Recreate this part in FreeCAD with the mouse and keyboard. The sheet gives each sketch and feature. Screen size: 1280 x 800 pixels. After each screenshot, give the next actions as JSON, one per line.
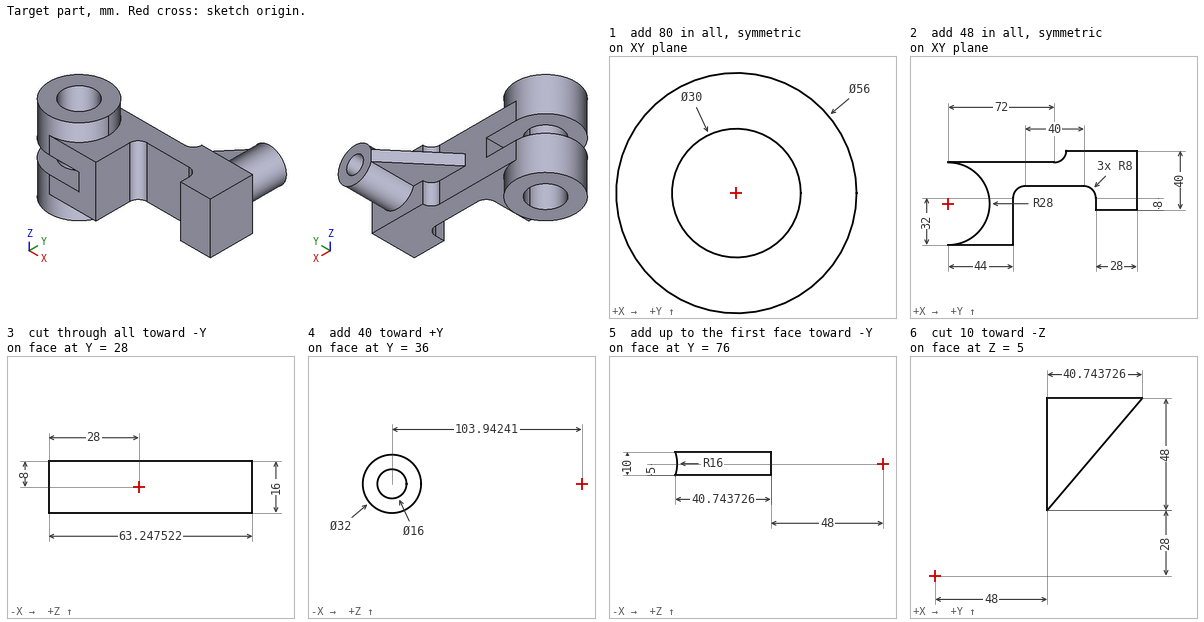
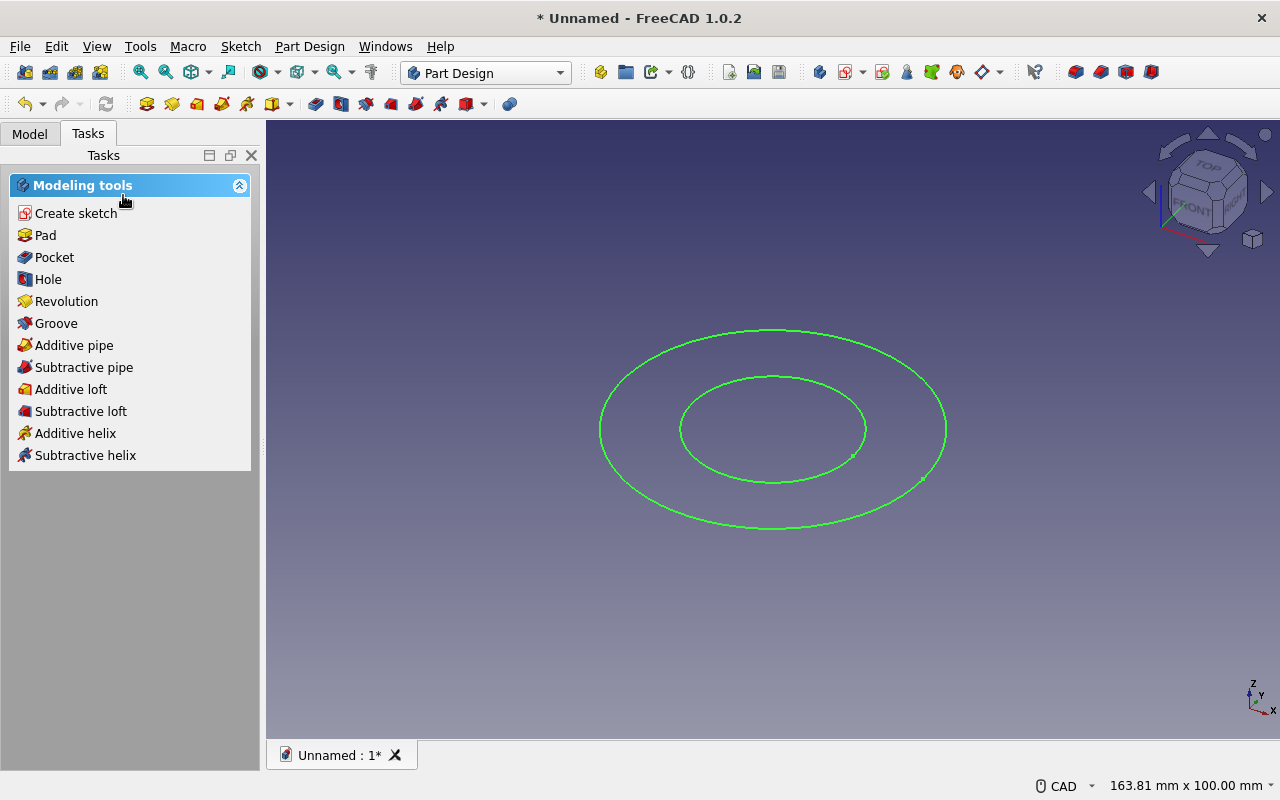
{"action": "left_click", "coordinate": [147, 104]}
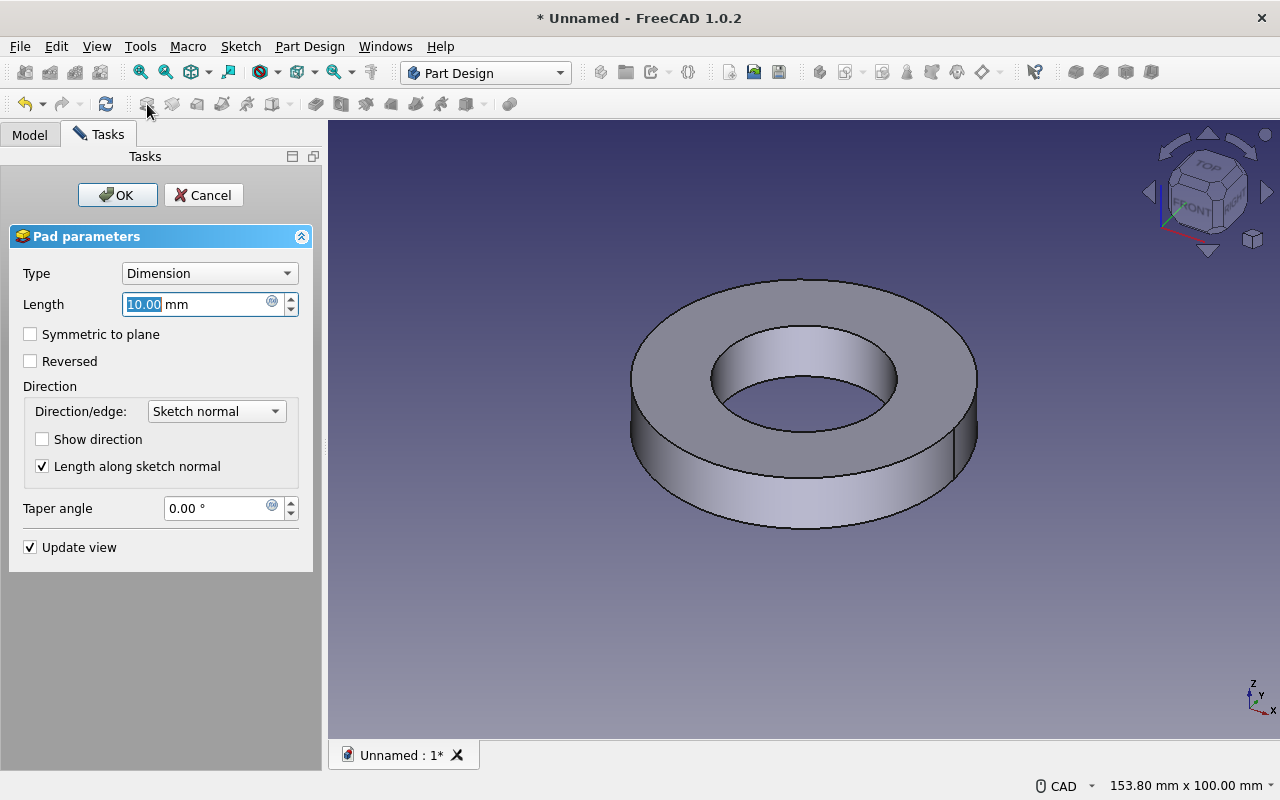
{"action": "type", "text": "80"}
{"action": "key", "text": "Tab"}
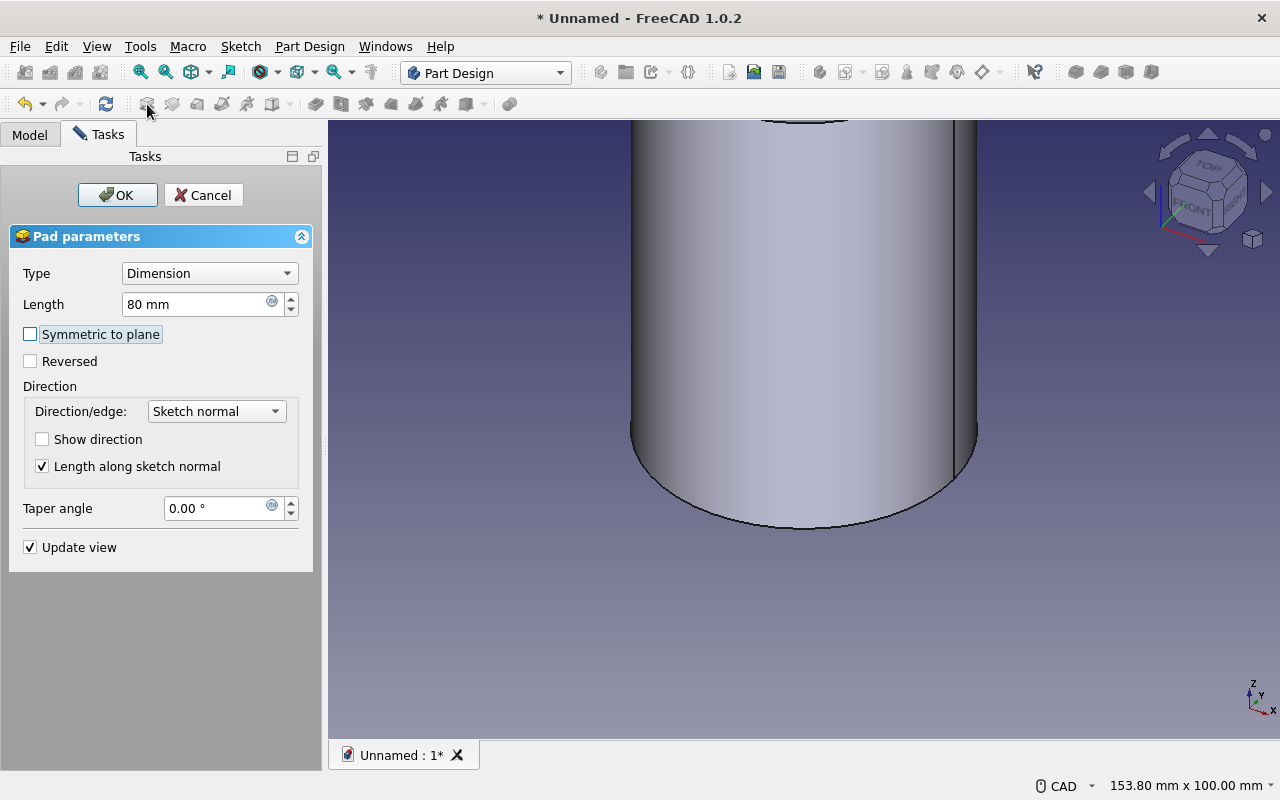
{"action": "left_click", "coordinate": [31, 334]}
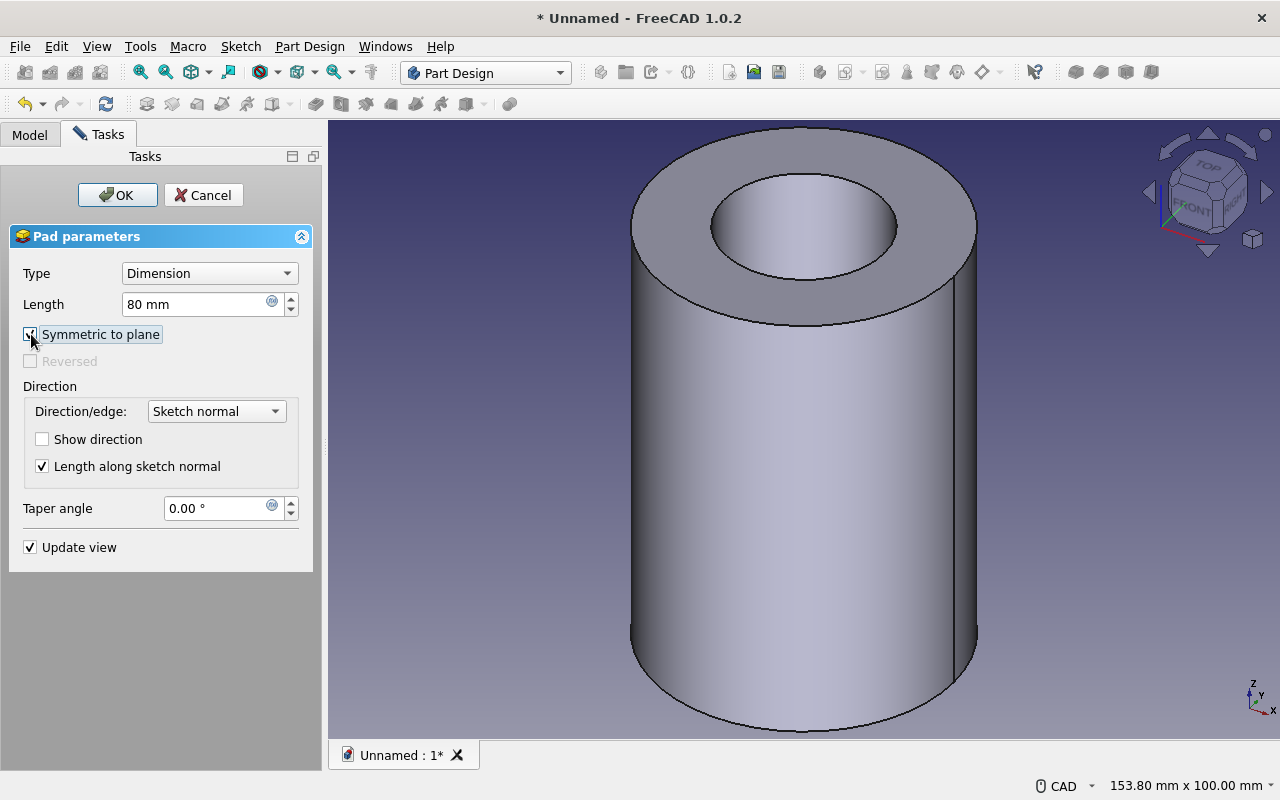
{"action": "left_click", "coordinate": [118, 195]}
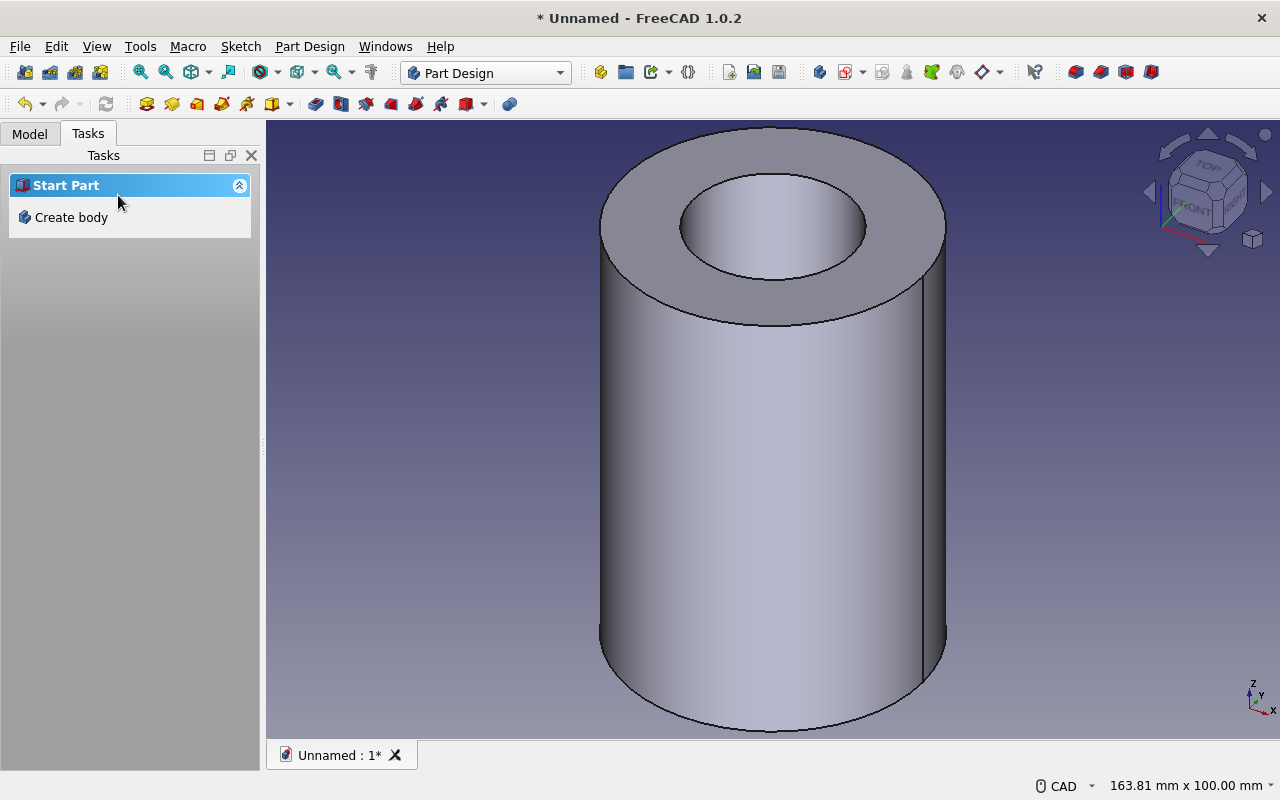
{"action": "key", "text": "v f"}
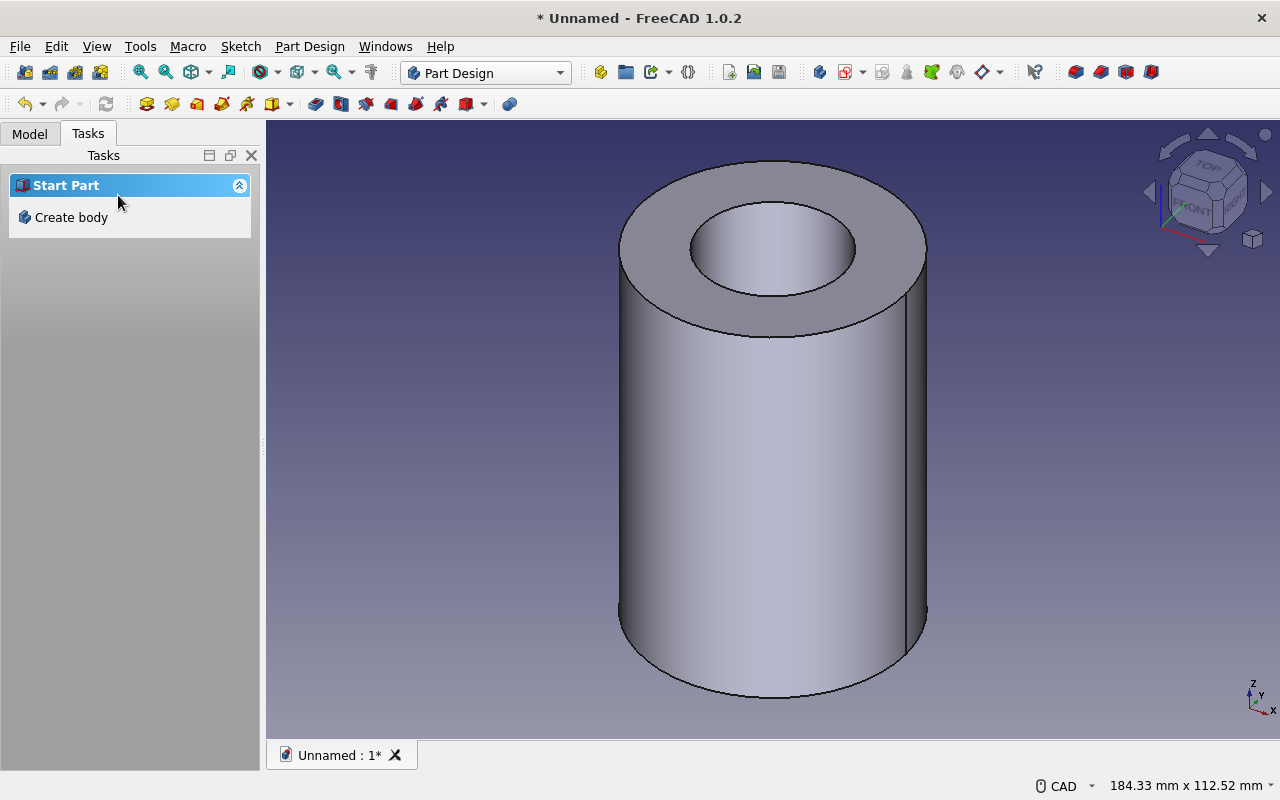
{"action": "left_click", "coordinate": [844, 72]}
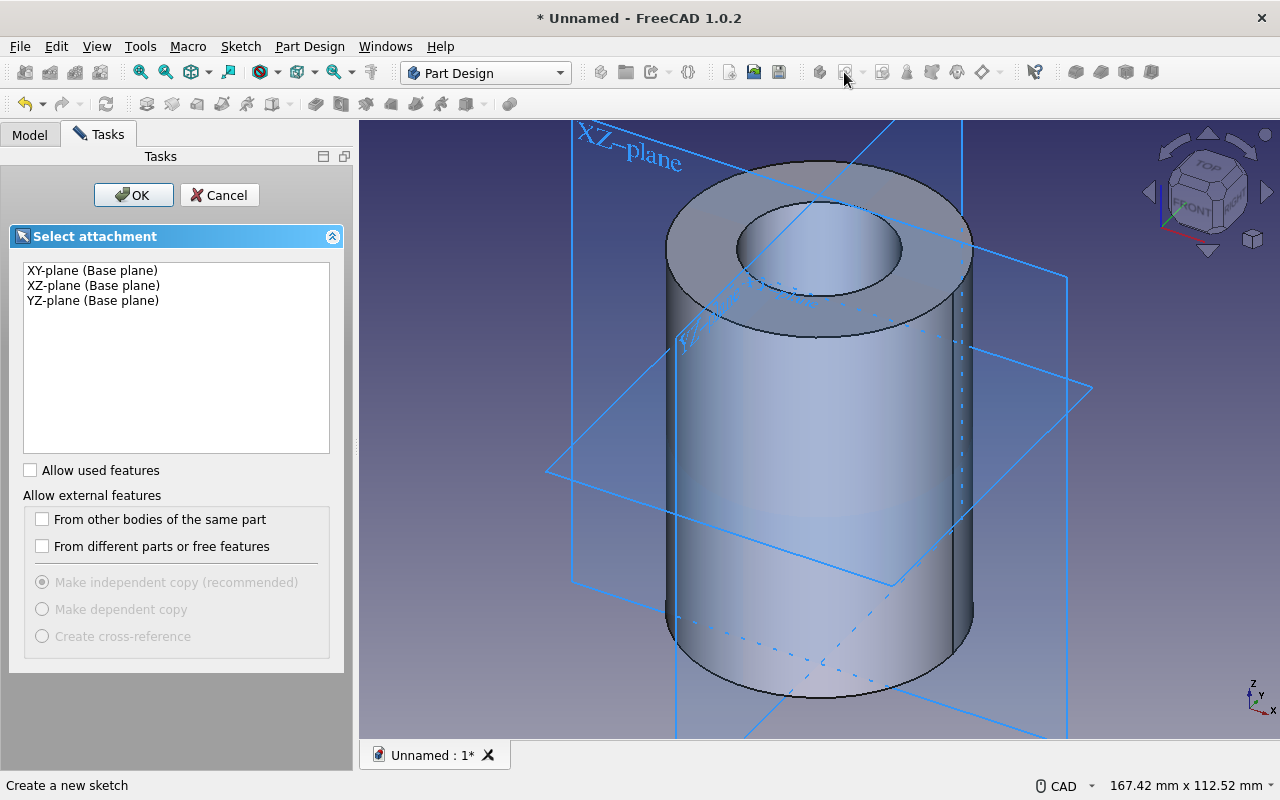
{"action": "left_click", "coordinate": [84, 270]}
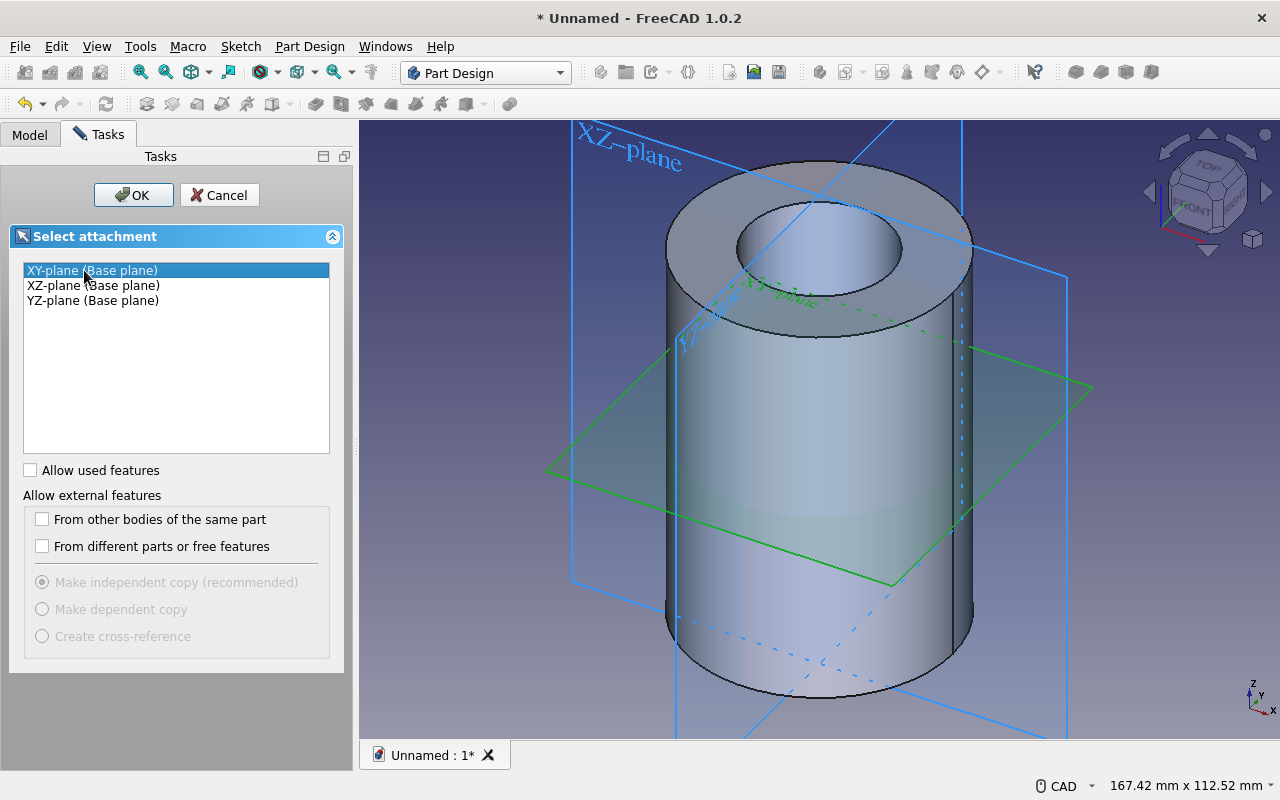
{"action": "left_click", "coordinate": [134, 195]}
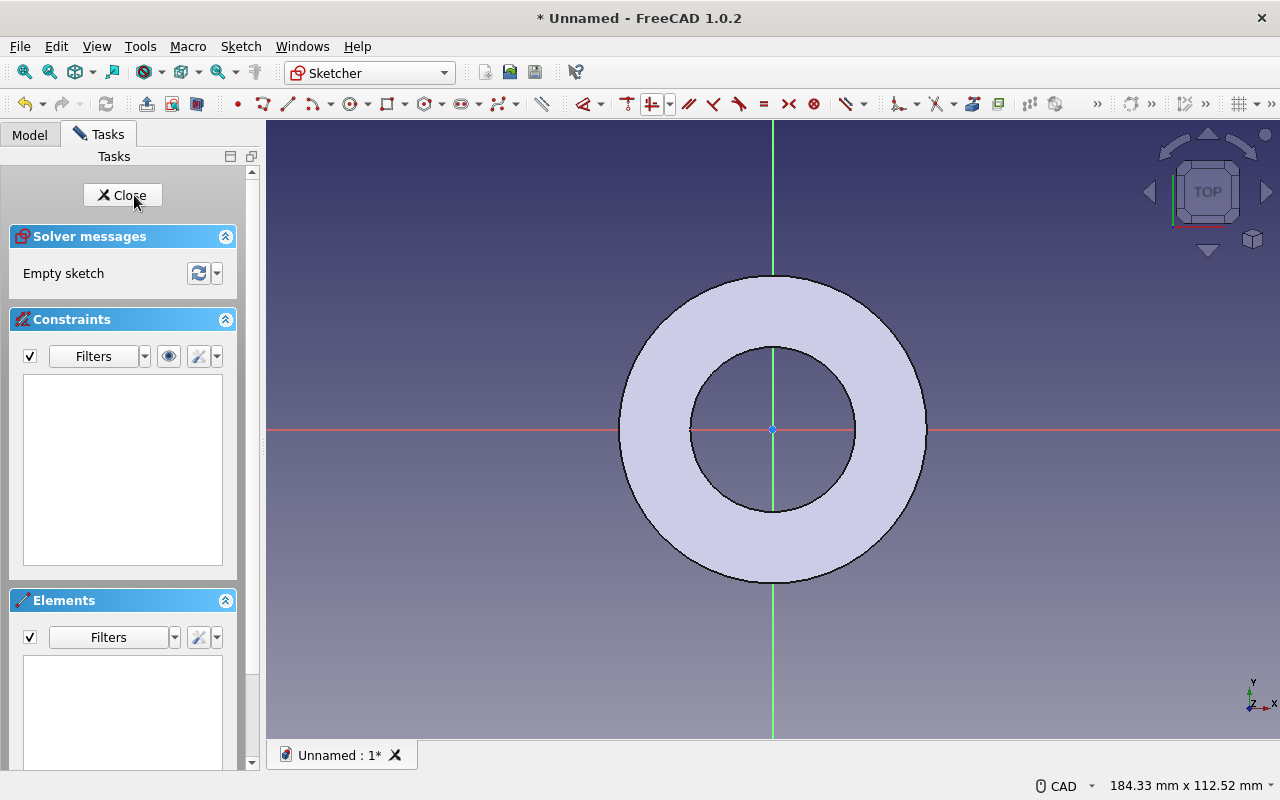
{"action": "key", "text": "q s"}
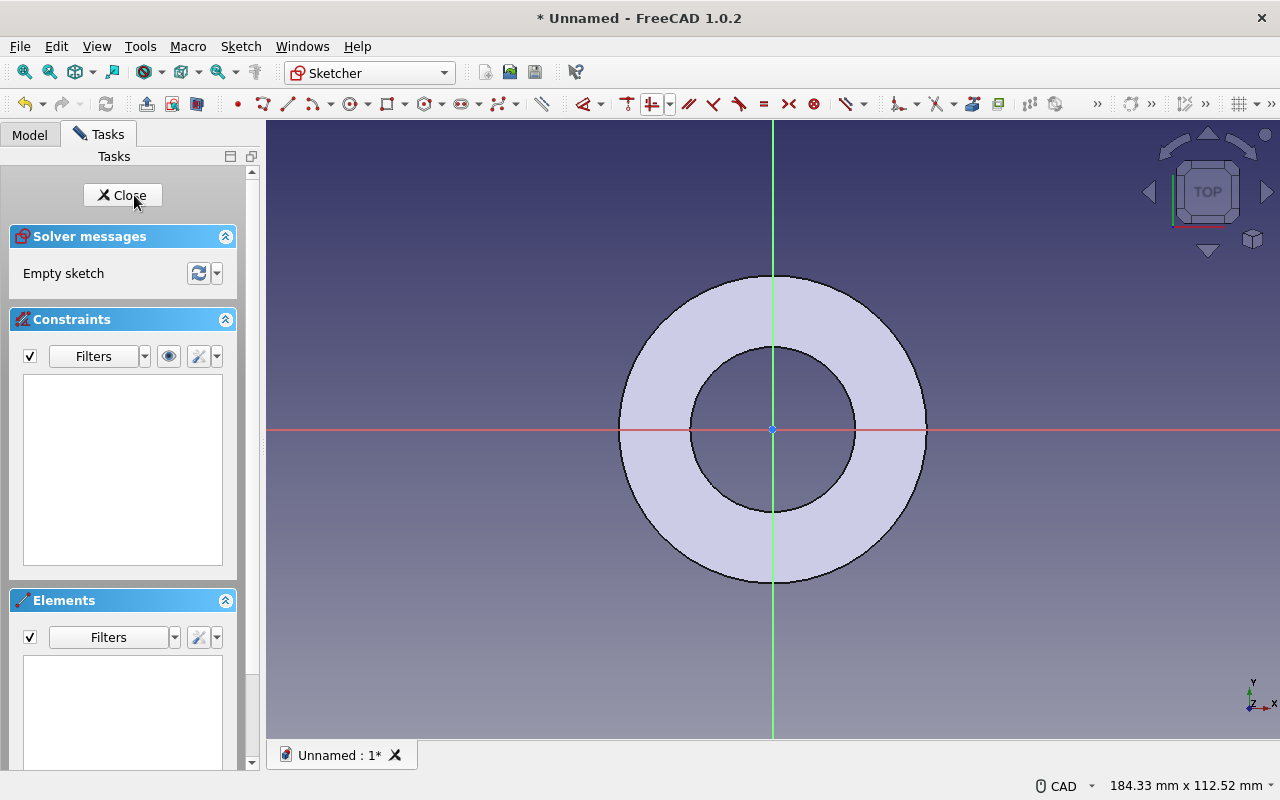
{"action": "scroll", "coordinate": [294, 474], "scroll_direction": "down", "scroll_amount": 2}